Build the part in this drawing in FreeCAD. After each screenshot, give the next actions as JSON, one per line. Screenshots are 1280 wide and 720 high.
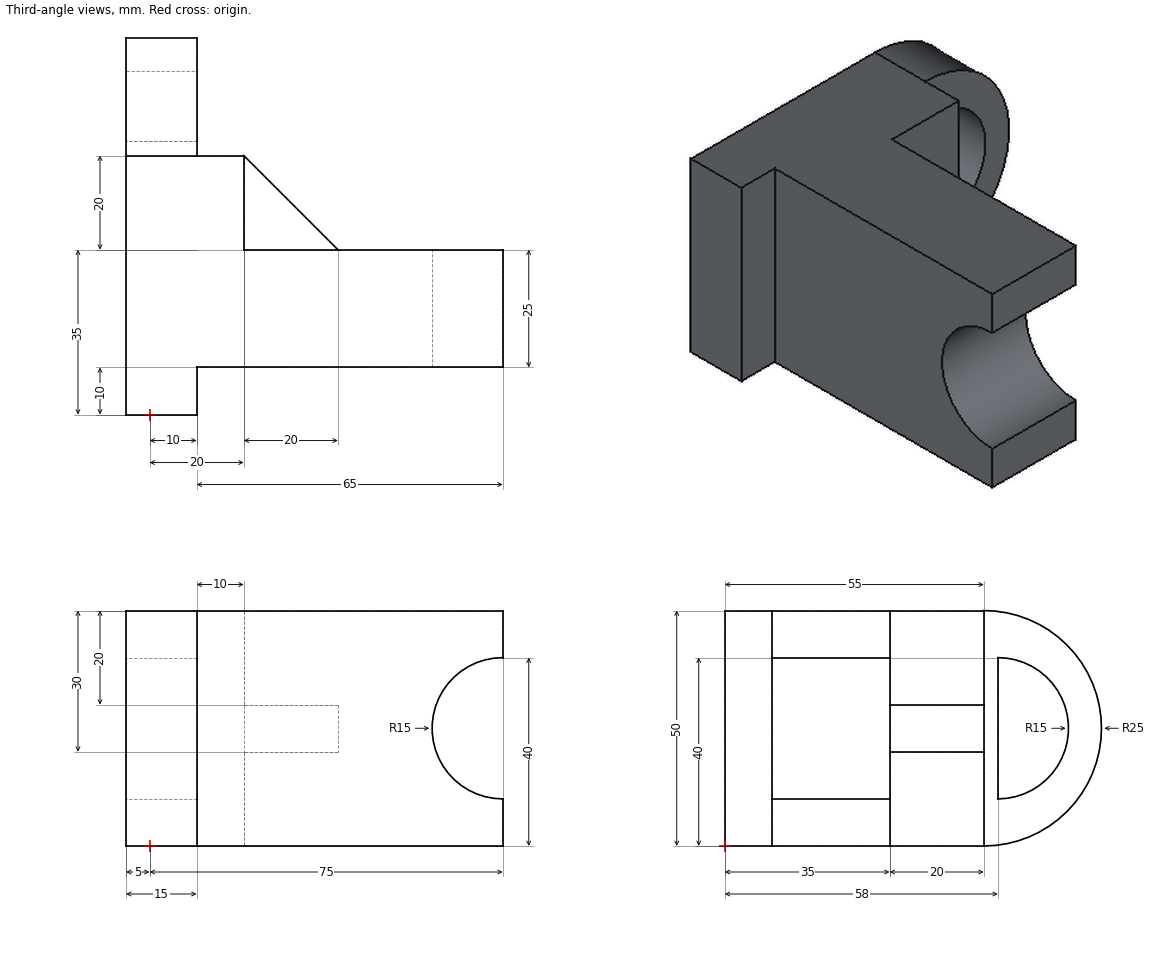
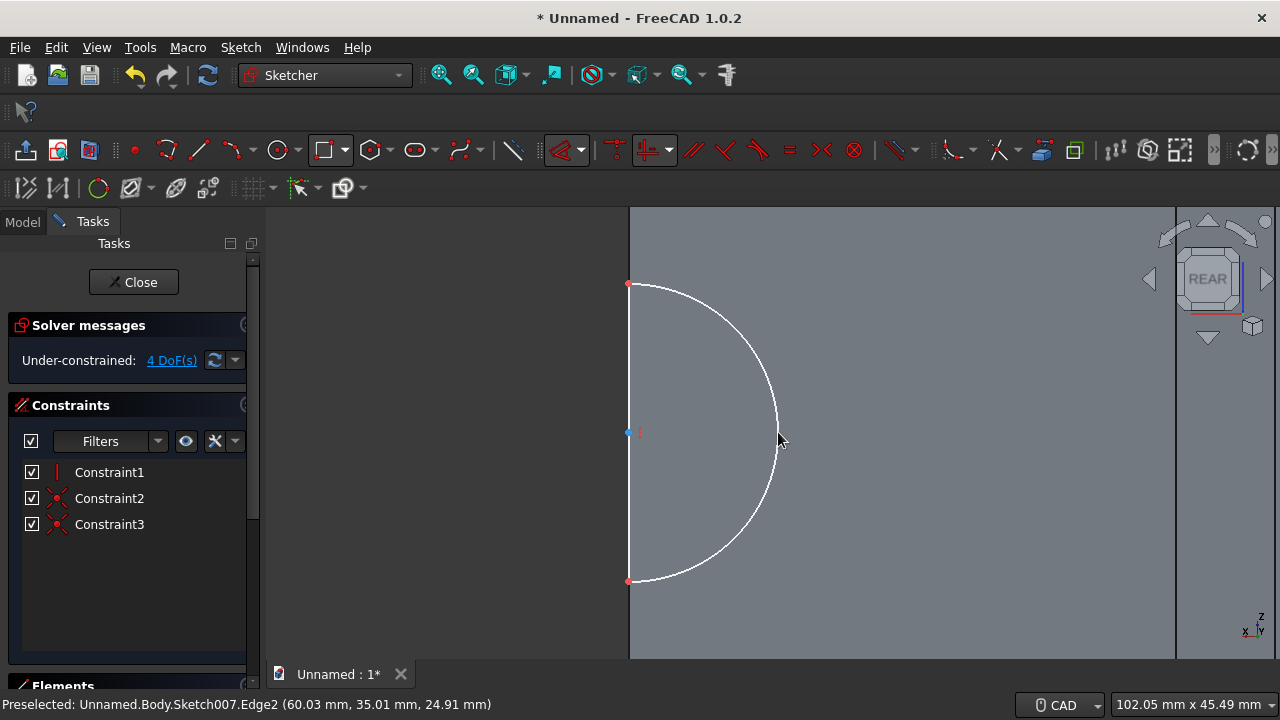
{"action": "left_click", "coordinate": [750, 521]}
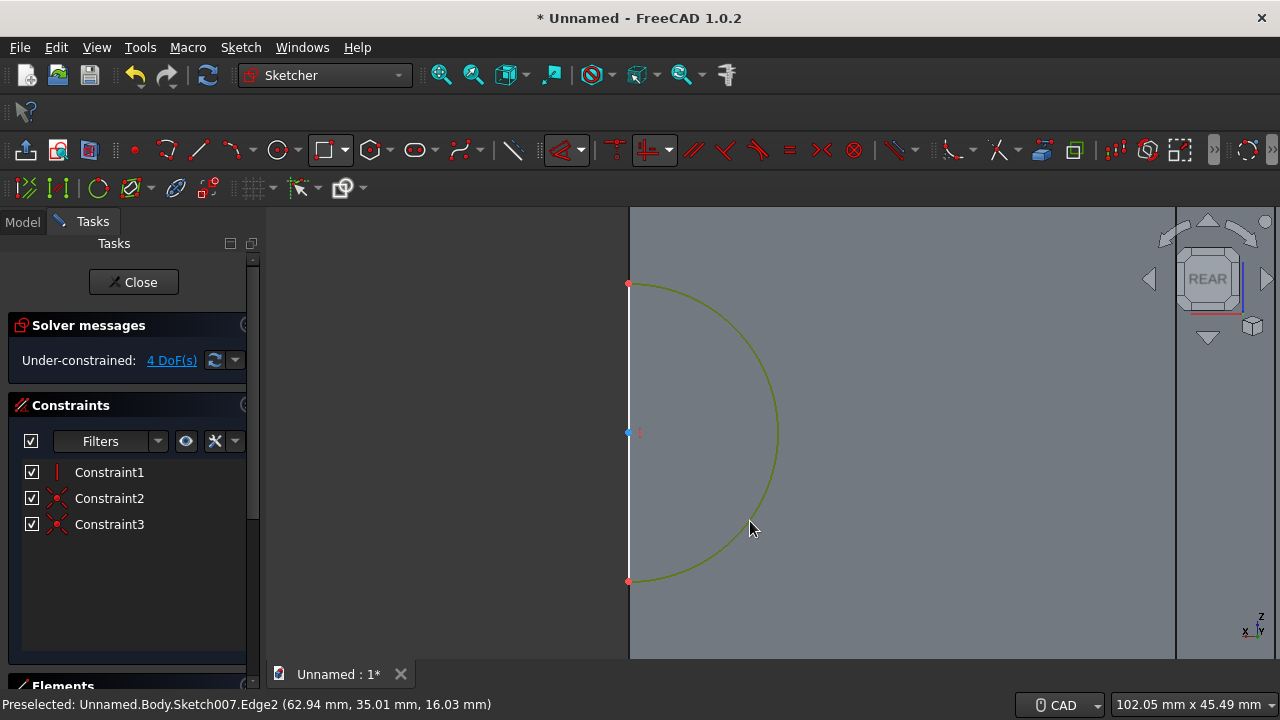
{"action": "left_click", "coordinate": [584, 150]}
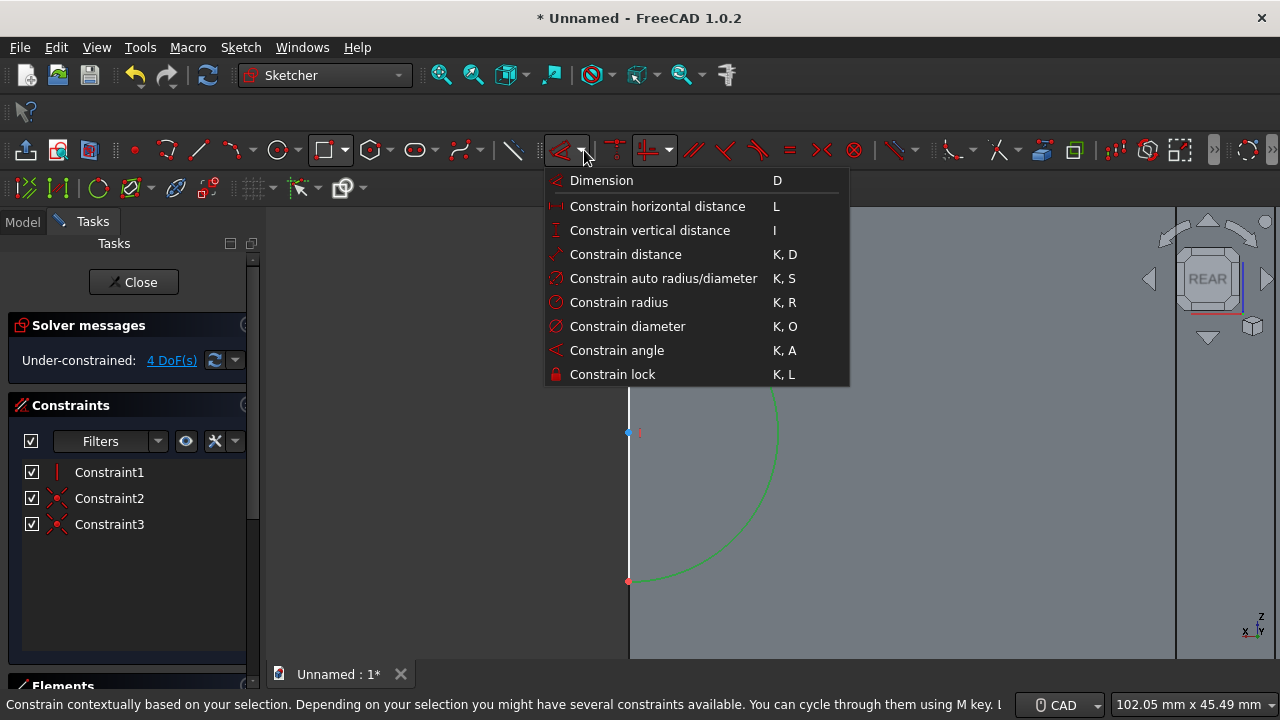
{"action": "left_click", "coordinate": [697, 302]}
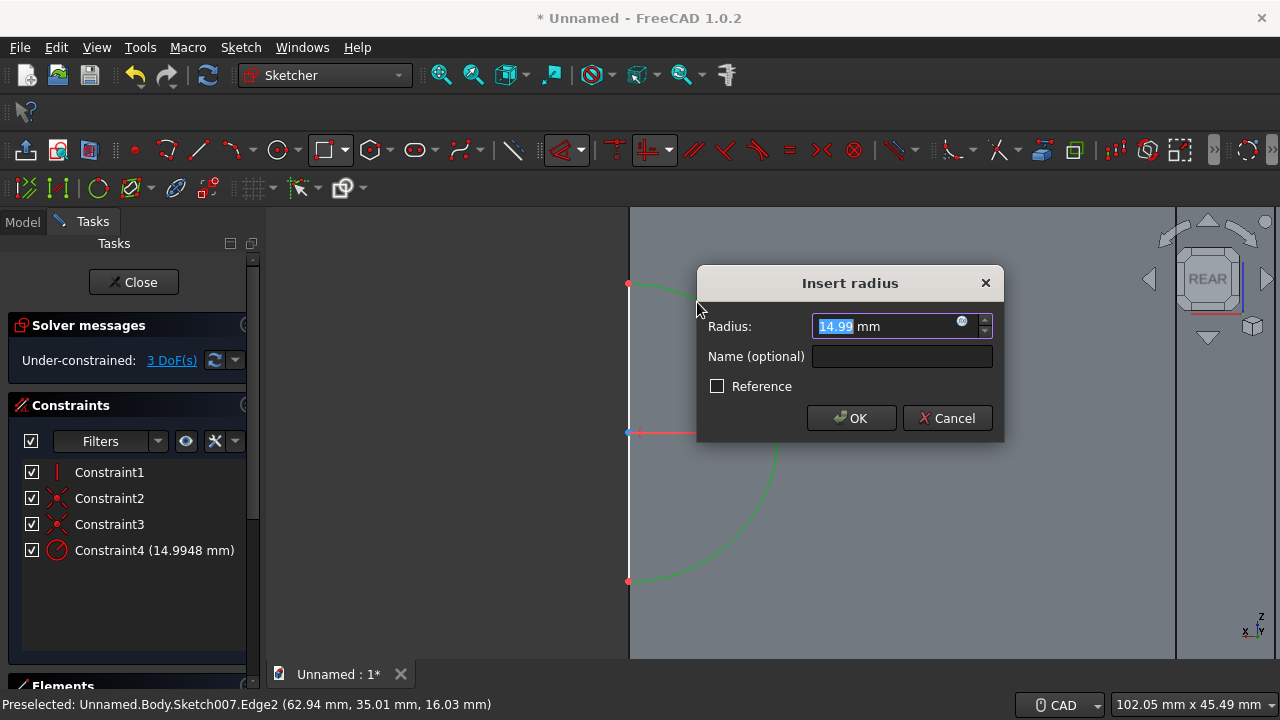
{"action": "type", "text": "15"}
{"action": "key", "text": "Return"}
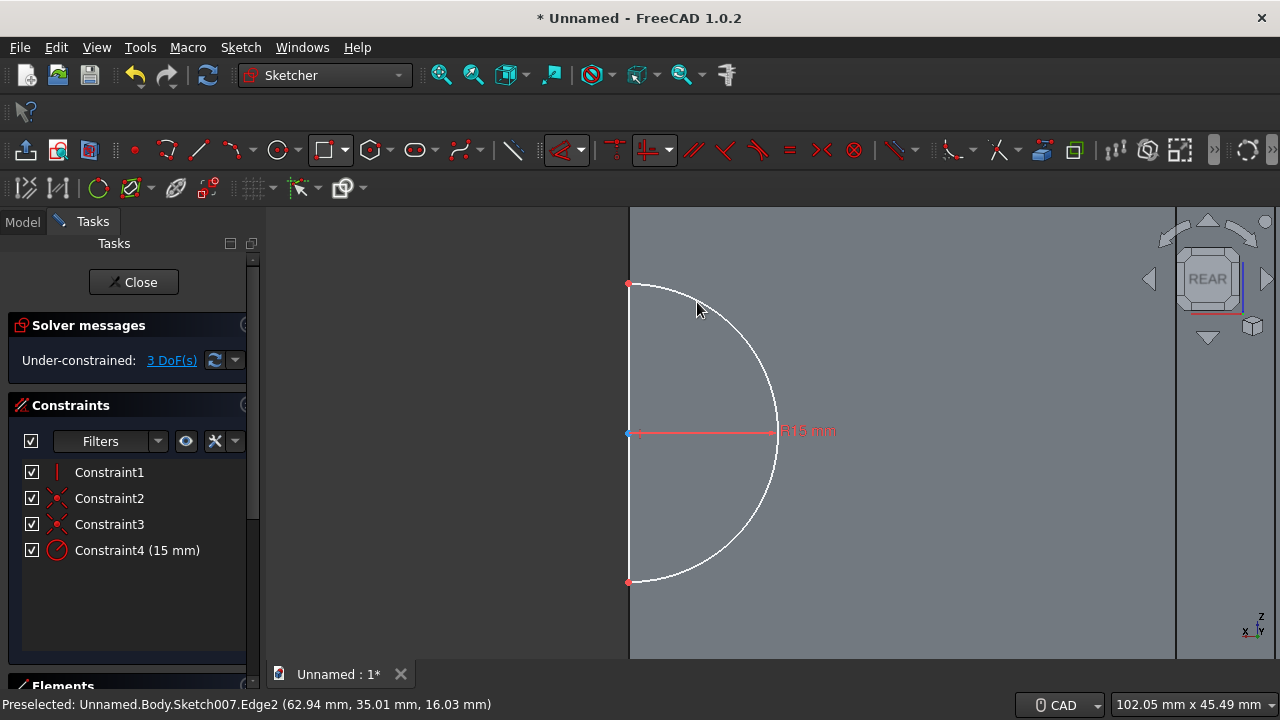
{"action": "left_click", "coordinate": [629, 284]}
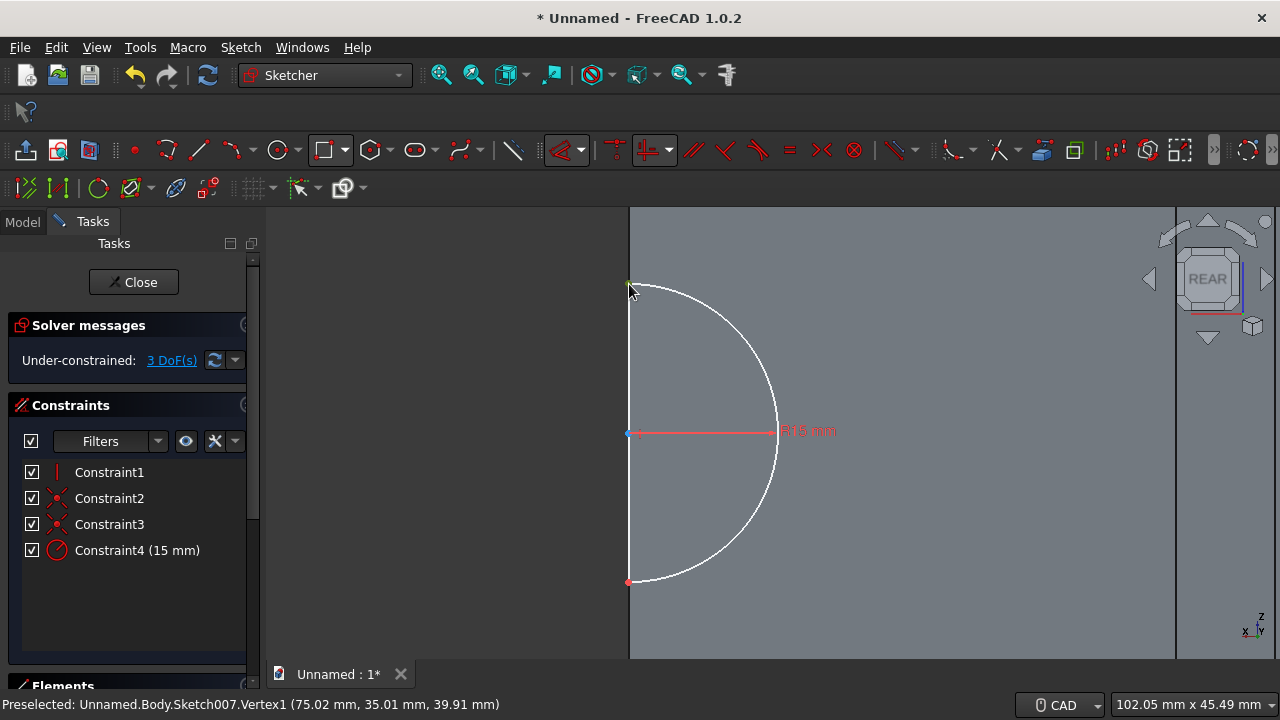
{"action": "left_click", "coordinate": [584, 150]}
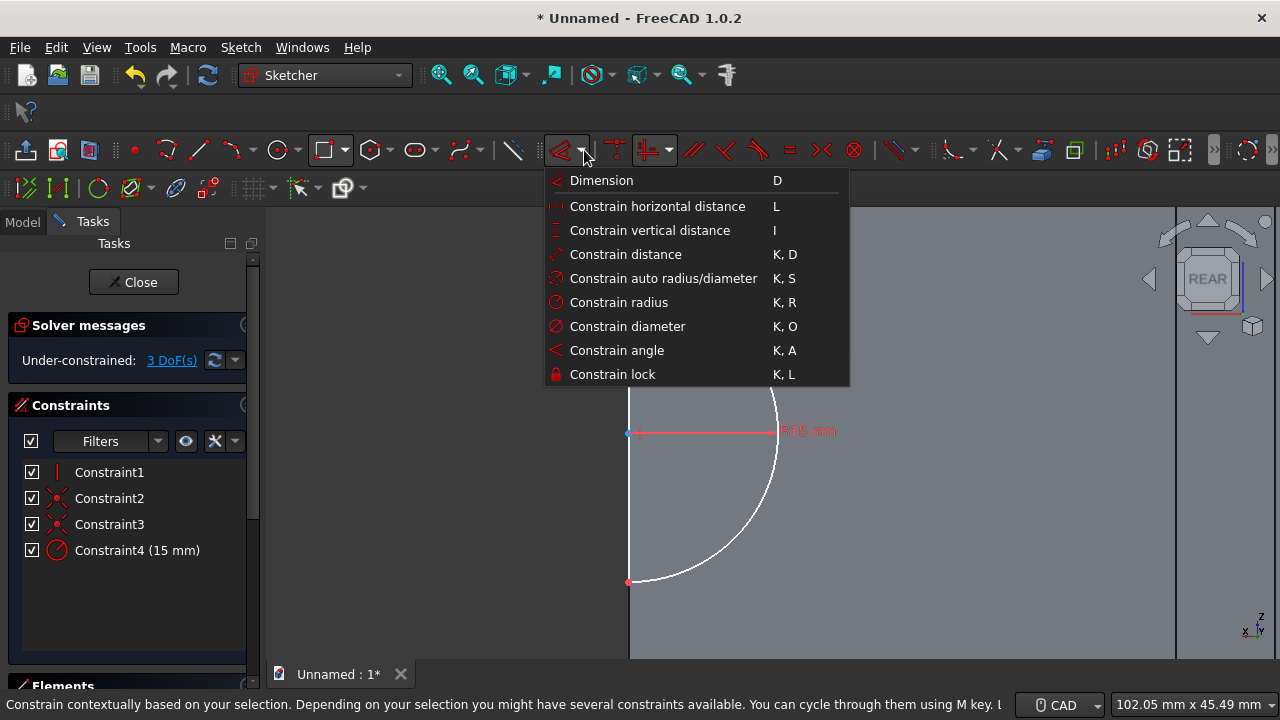
{"action": "left_click", "coordinate": [697, 206]}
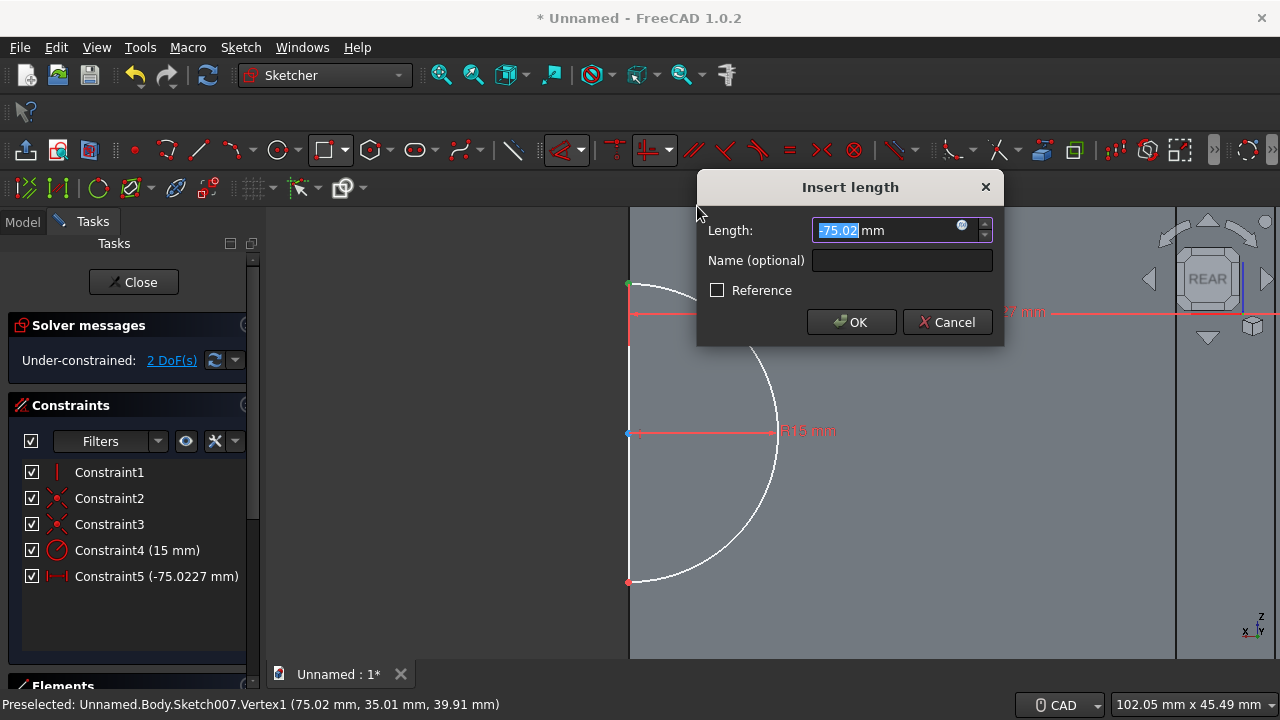
{"action": "type", "text": "-75"}
{"action": "key", "text": "Return"}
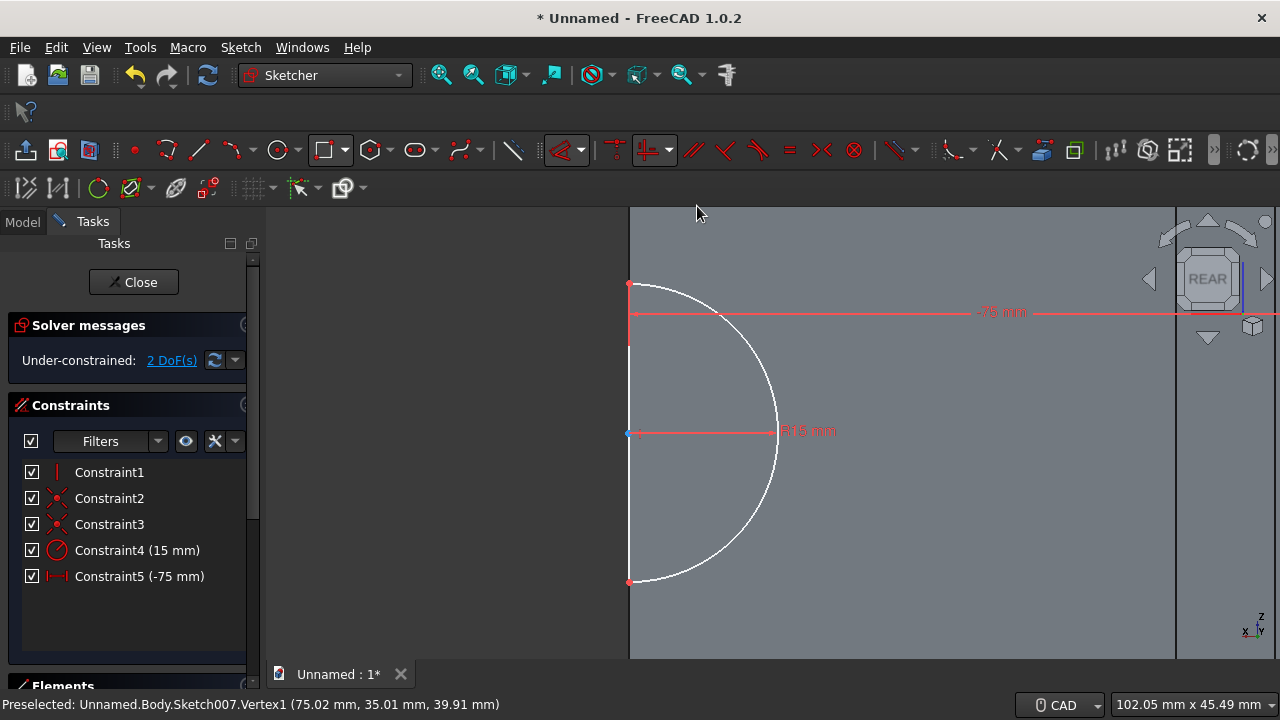
{"action": "left_click", "coordinate": [629, 284]}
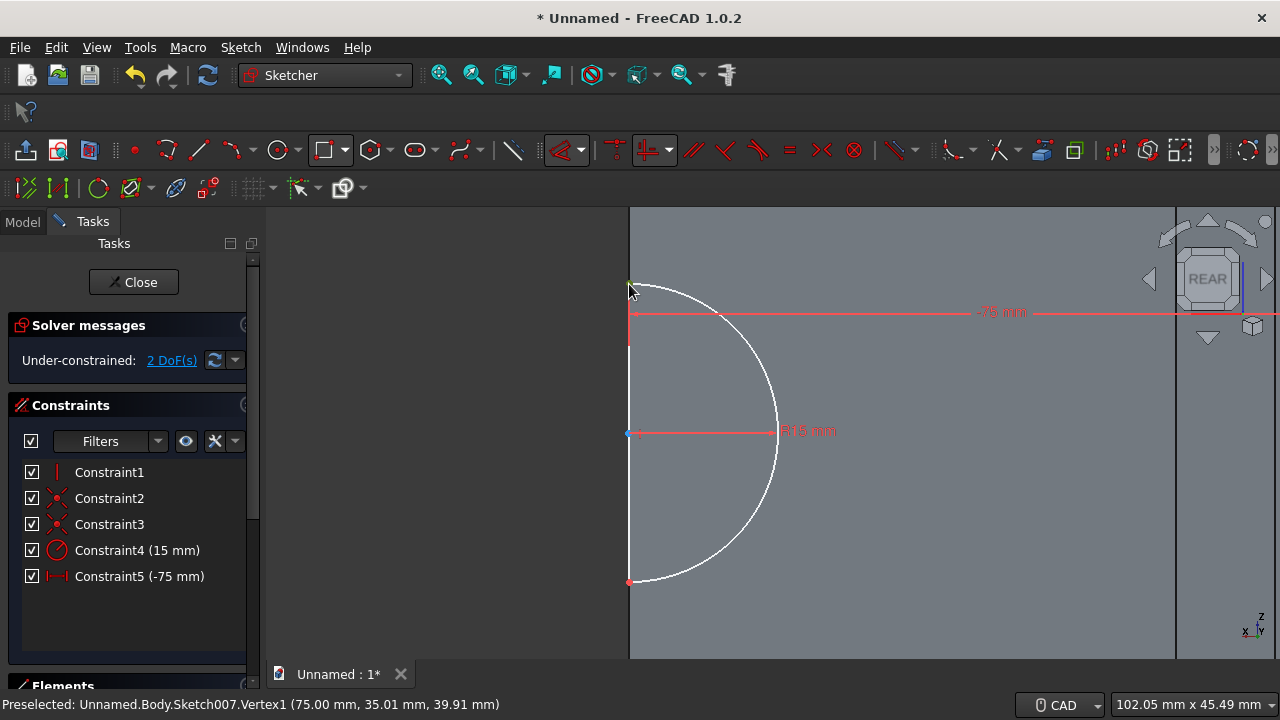
{"action": "key", "text": "i"}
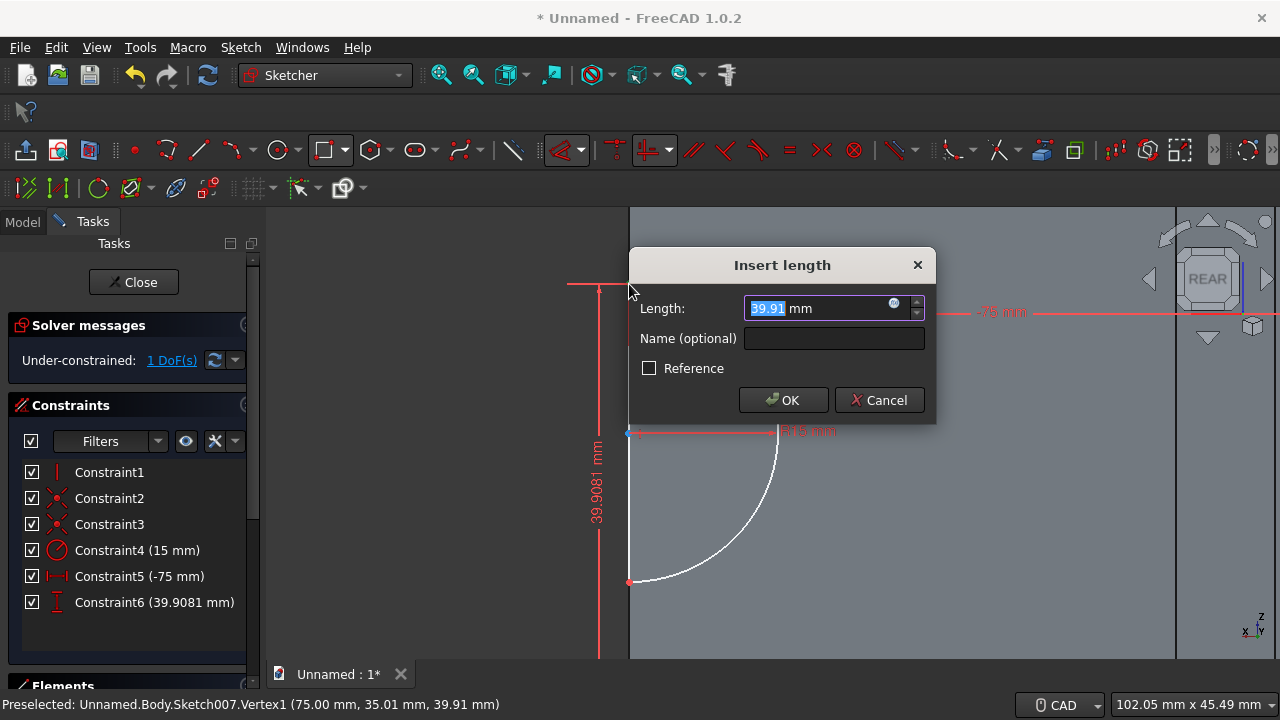
{"action": "type", "text": "40"}
{"action": "key", "text": "Return"}